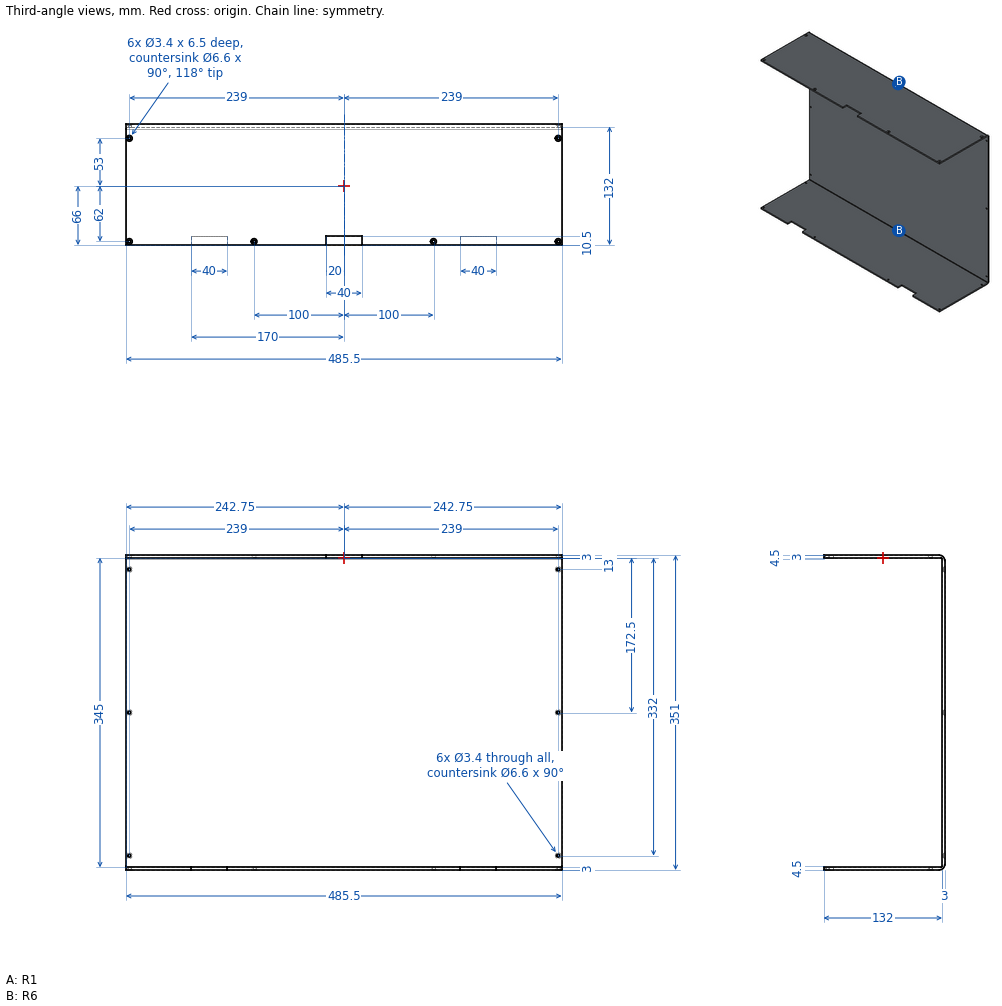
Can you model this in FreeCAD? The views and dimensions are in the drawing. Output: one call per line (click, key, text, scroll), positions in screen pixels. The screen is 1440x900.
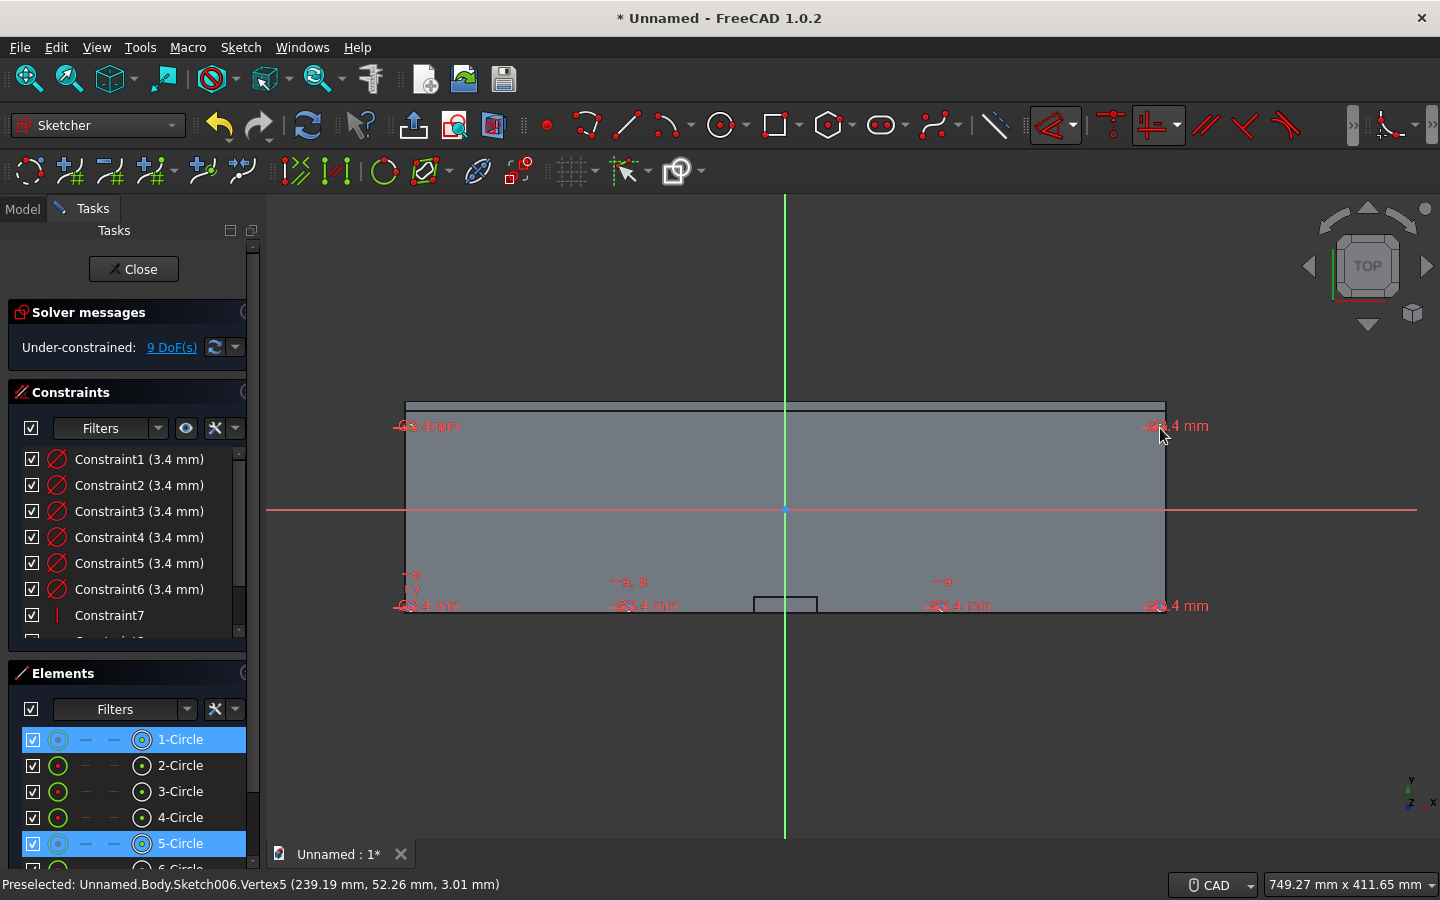
click(1180, 126)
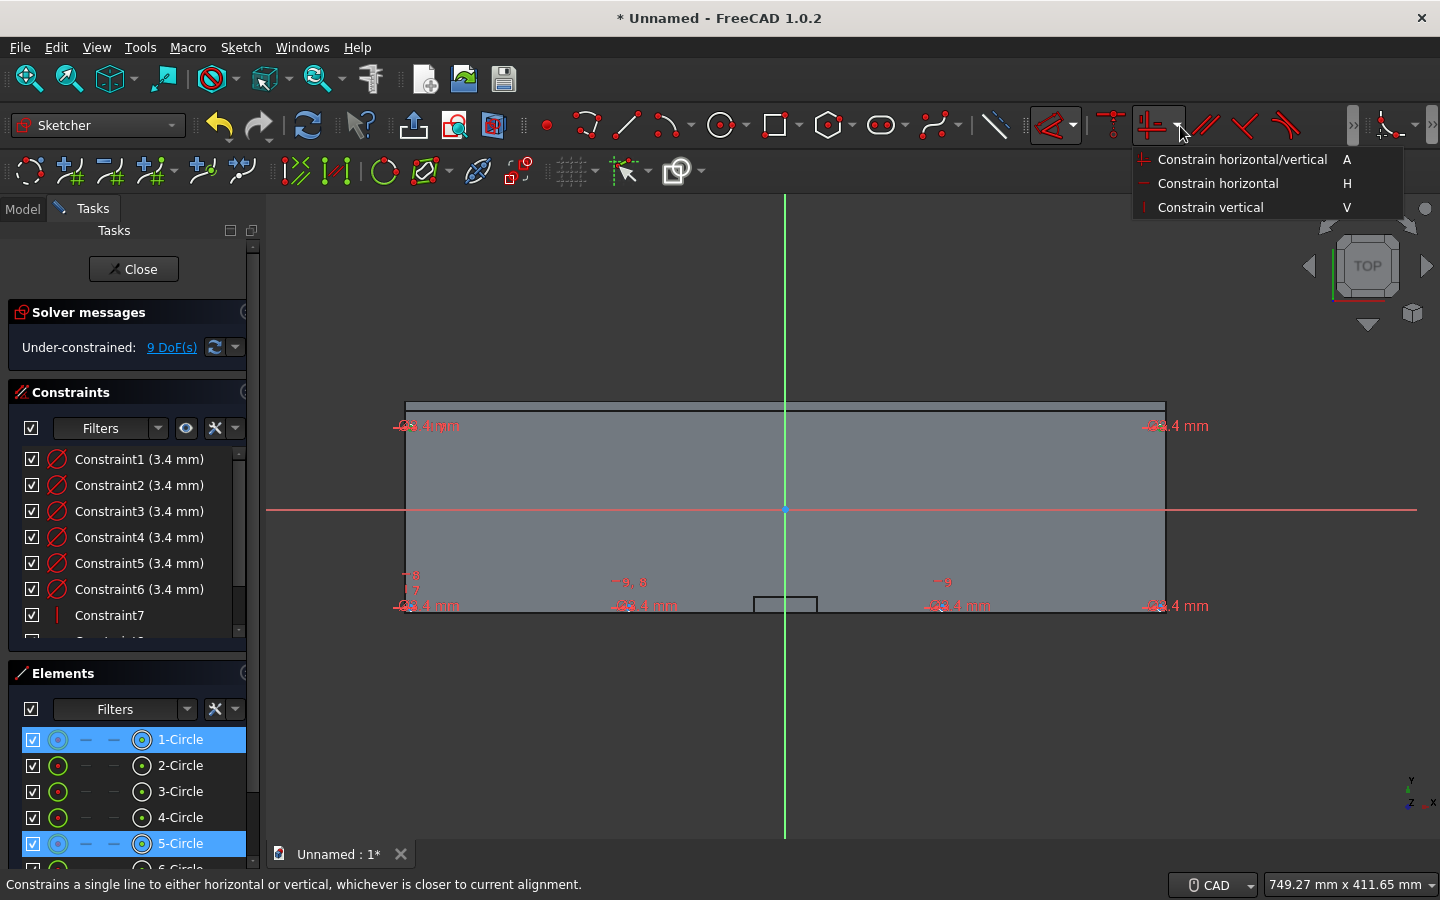
click(1268, 183)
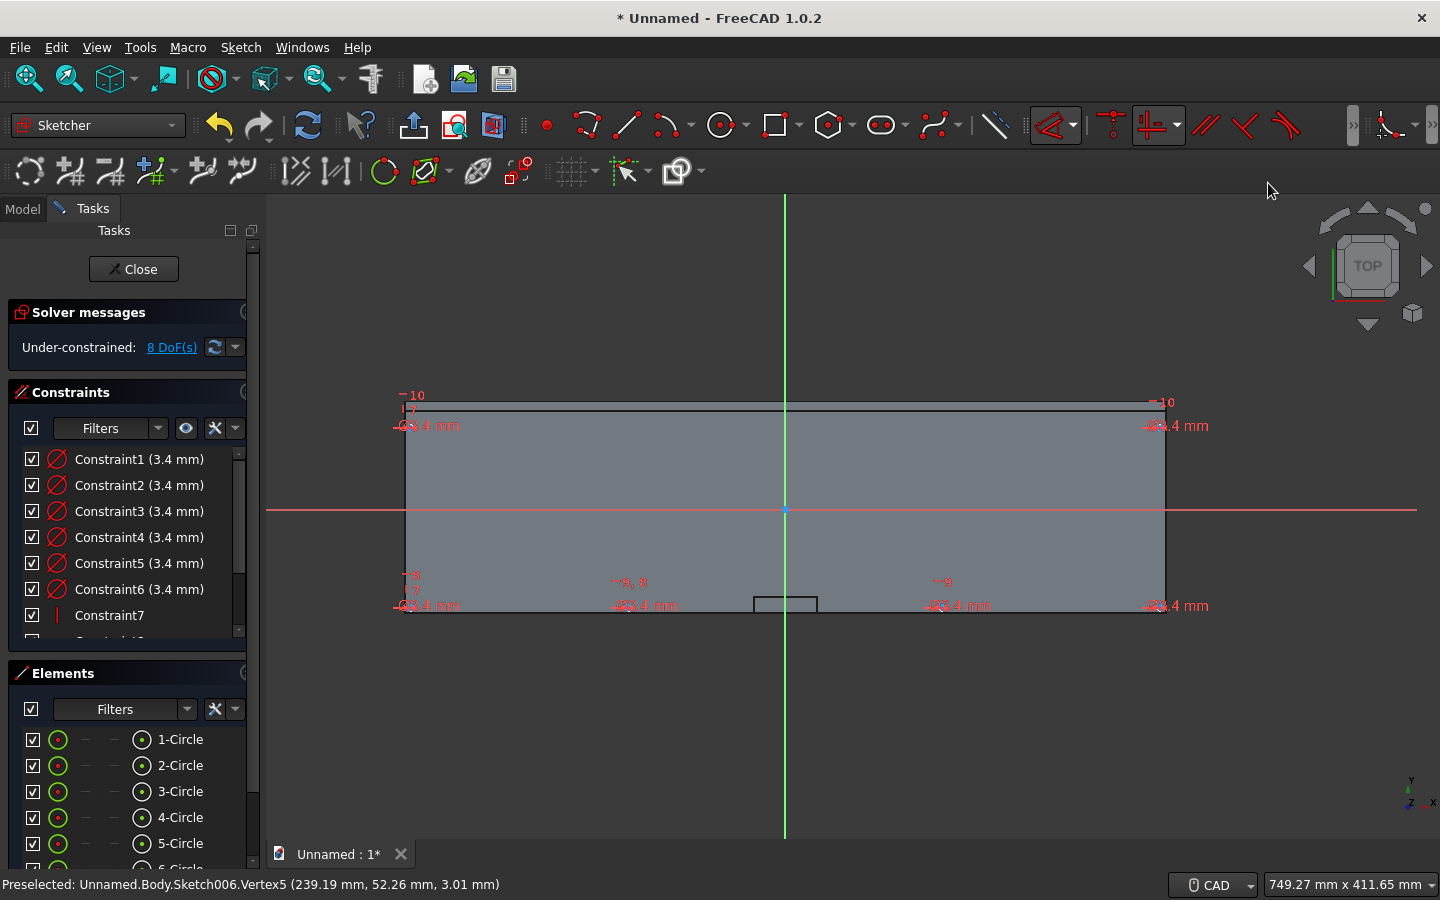
click(1160, 428)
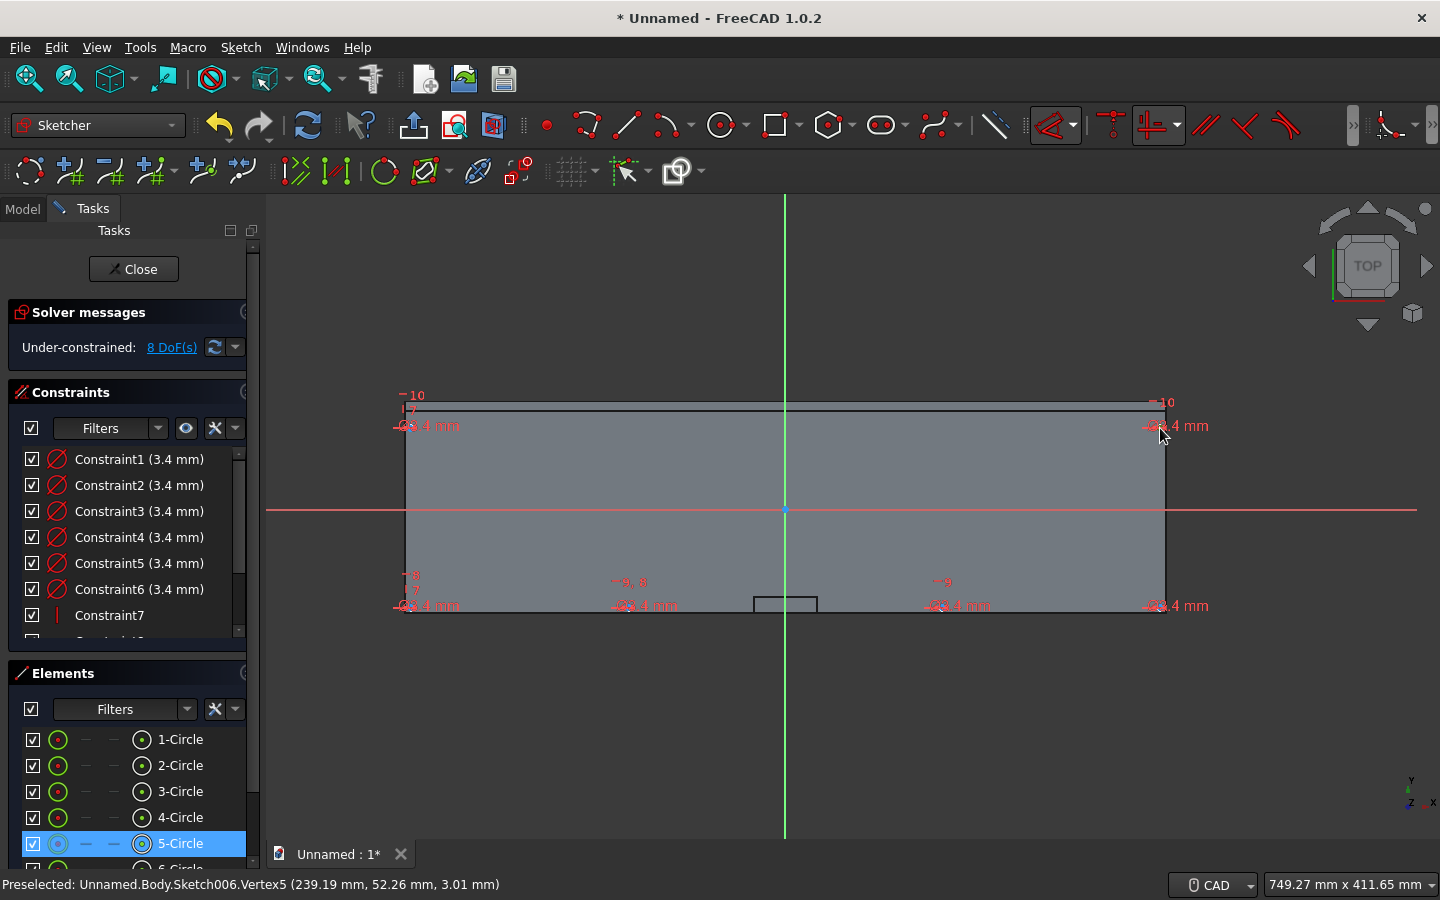
click(1160, 608)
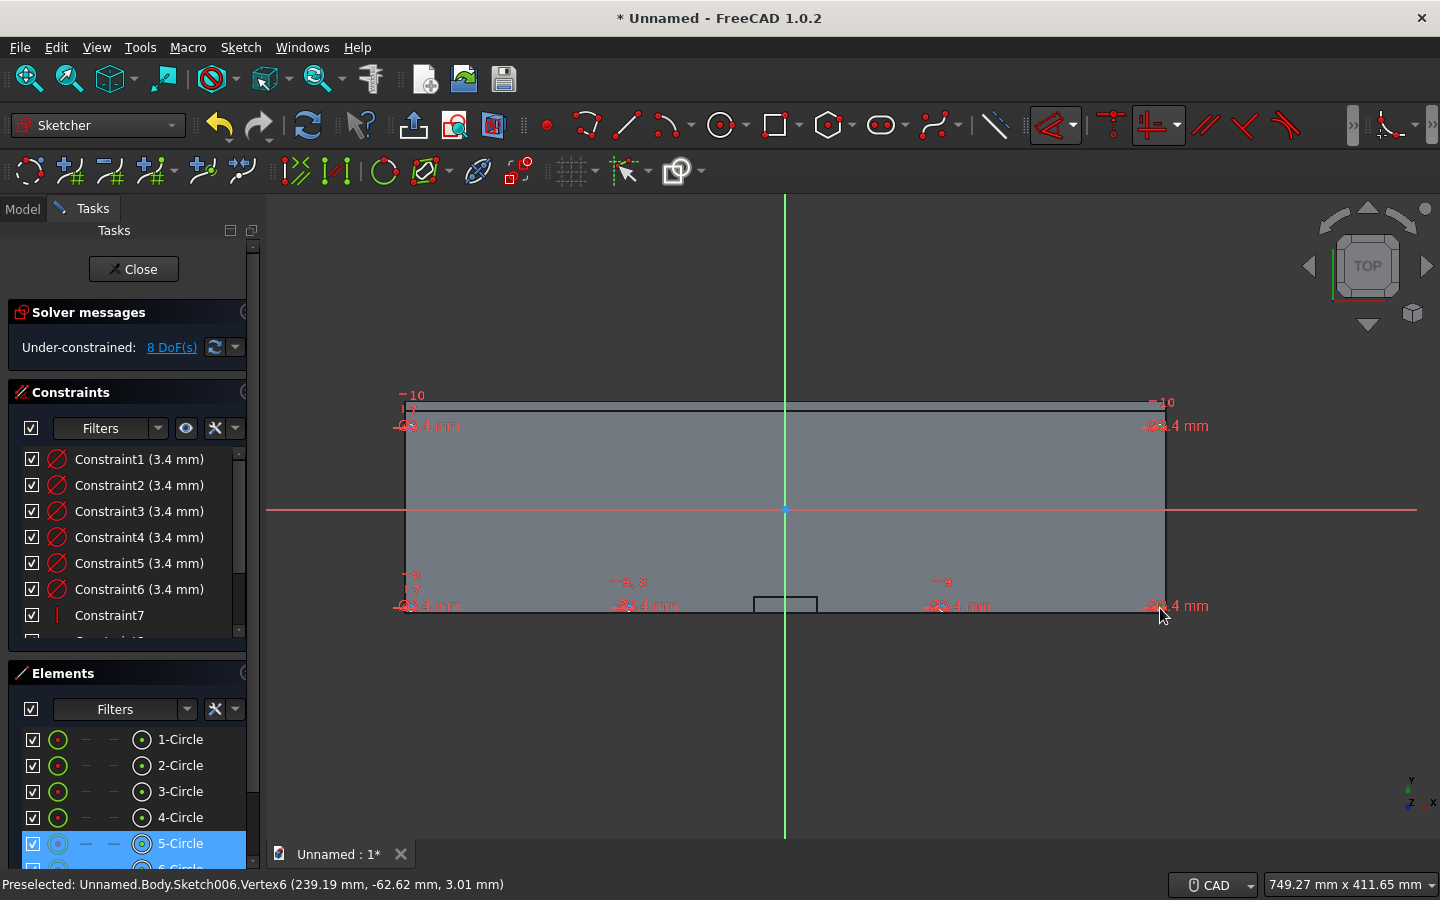
click(1180, 126)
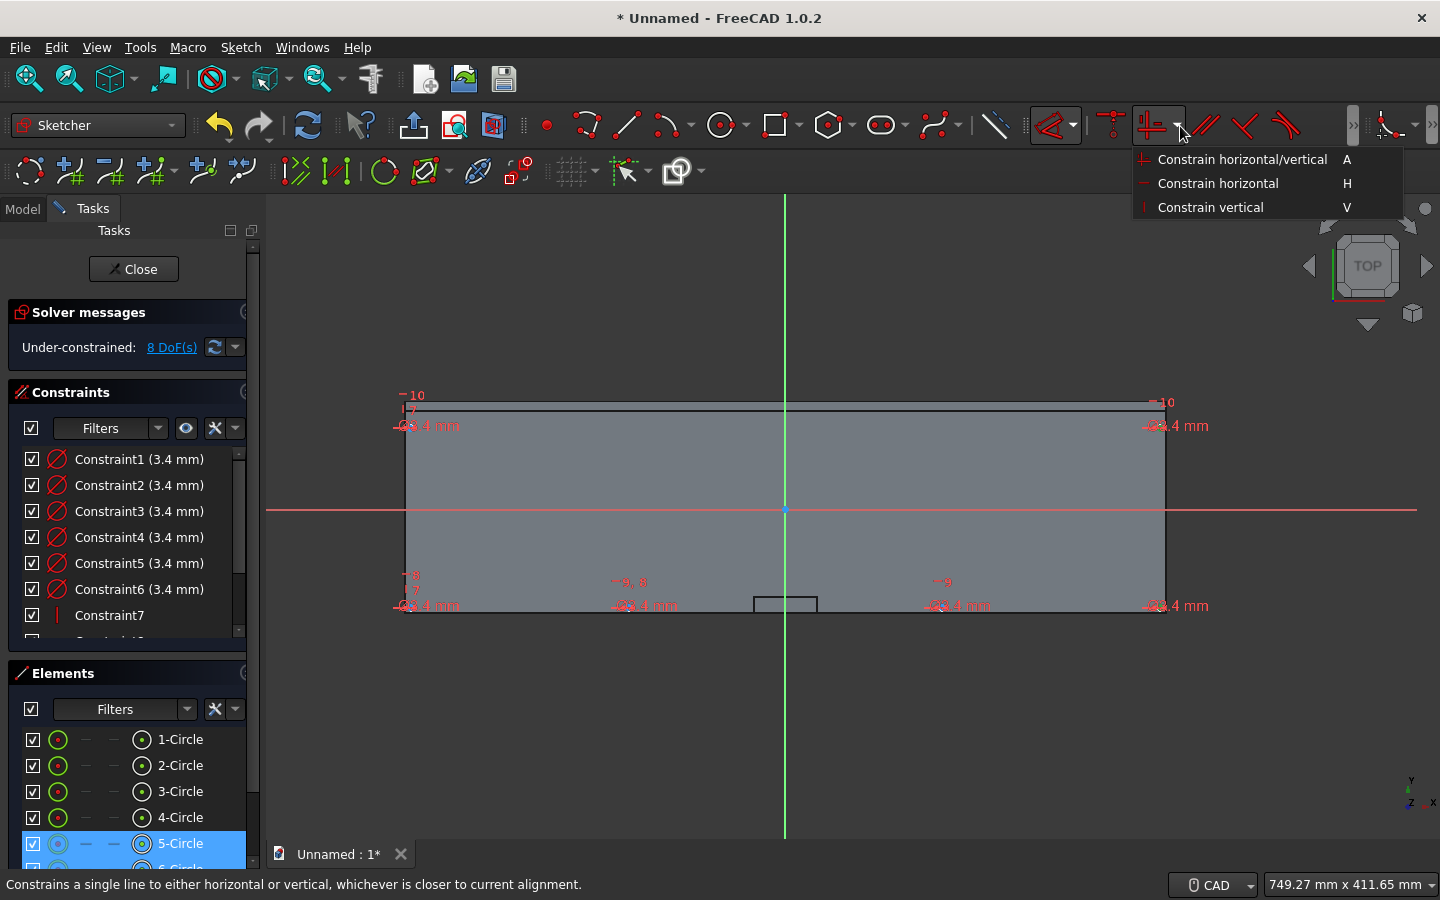
click(1268, 207)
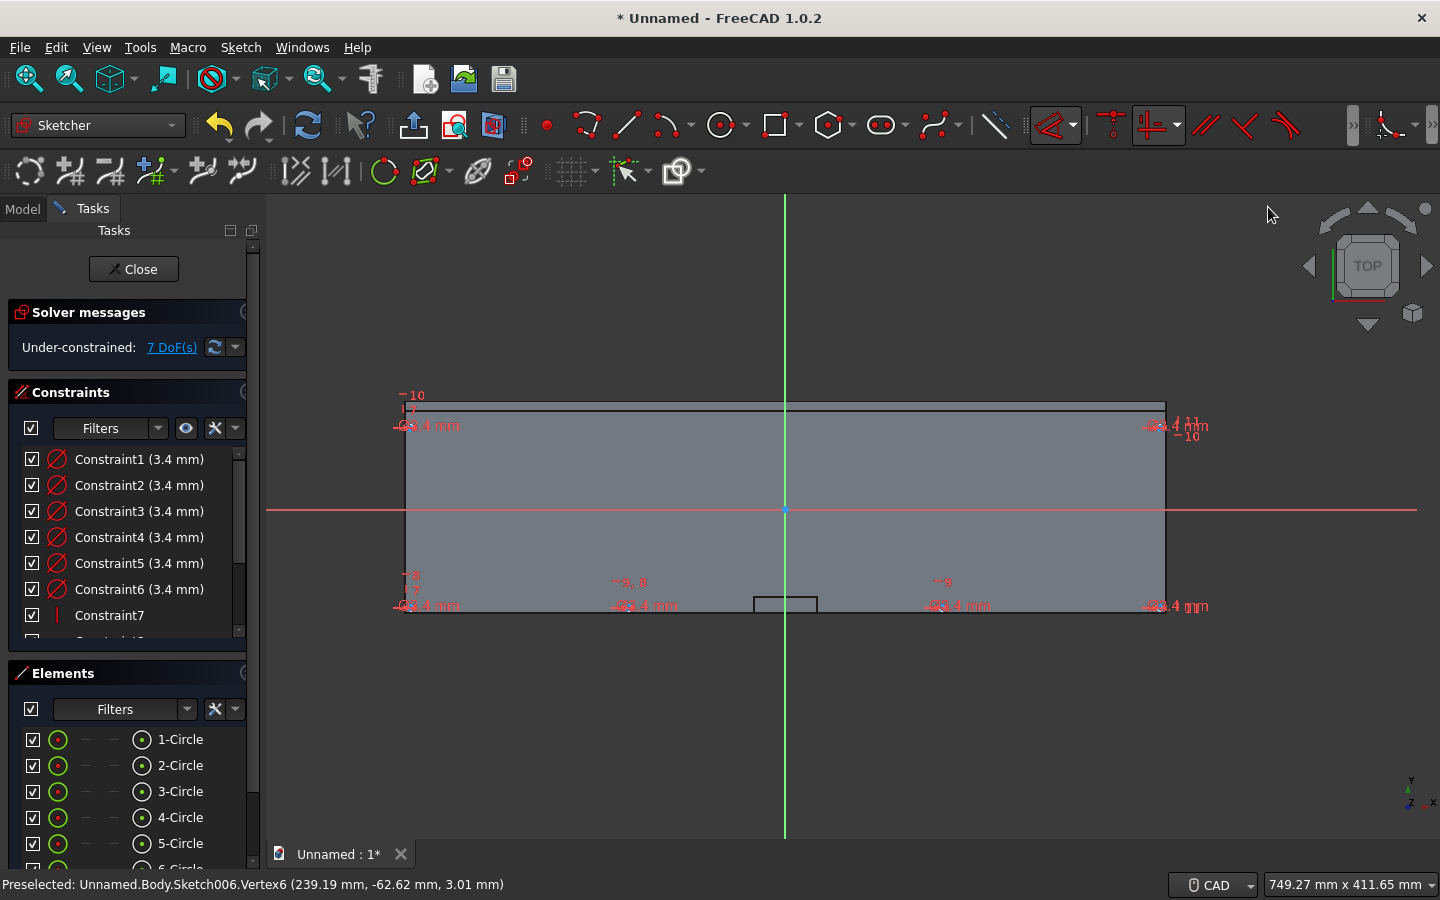
click(942, 608)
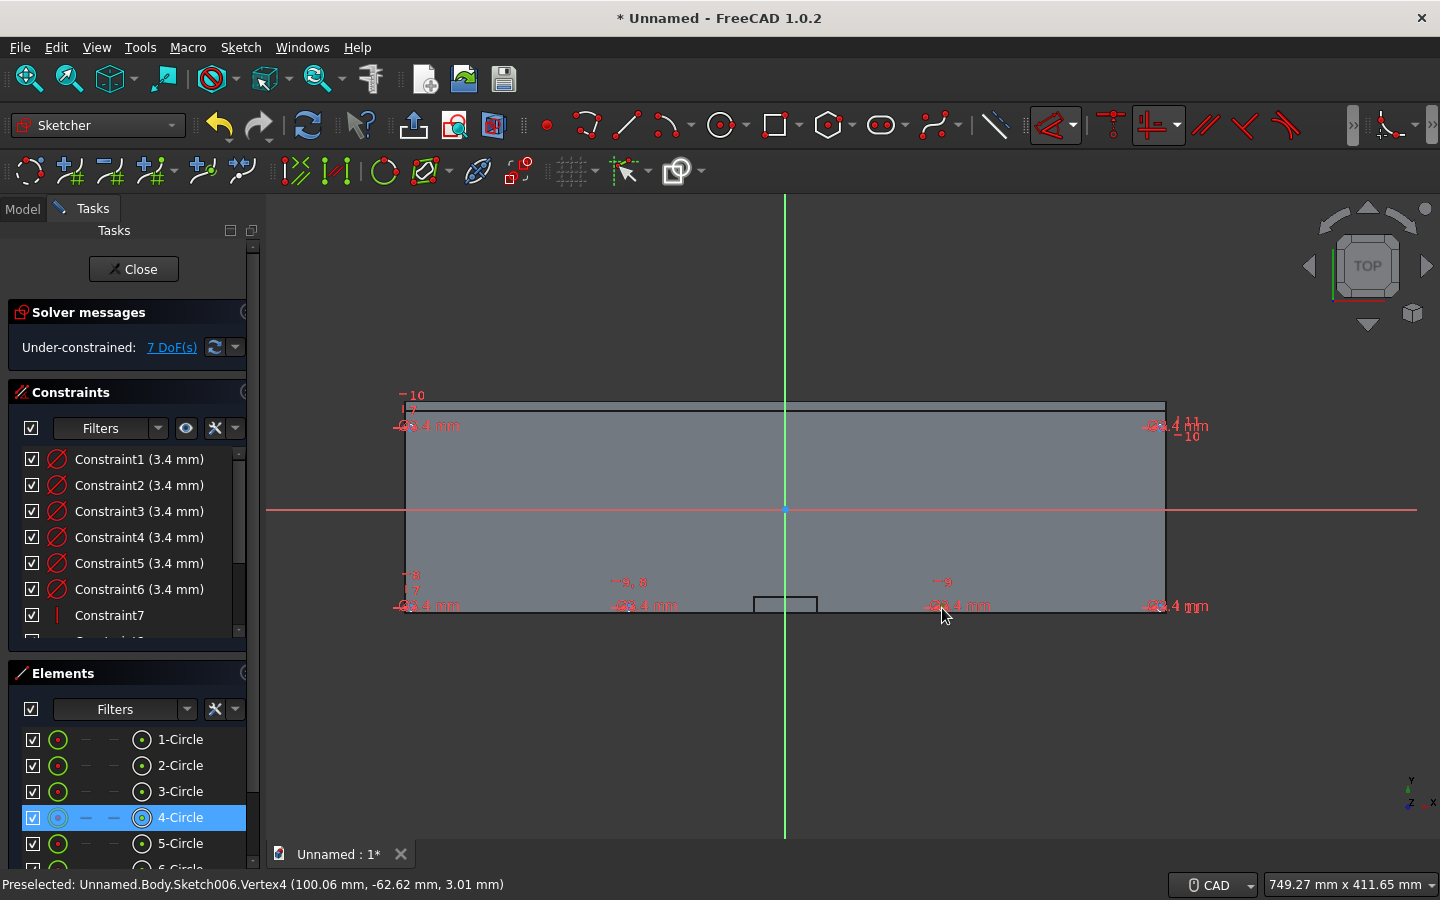
click(1160, 608)